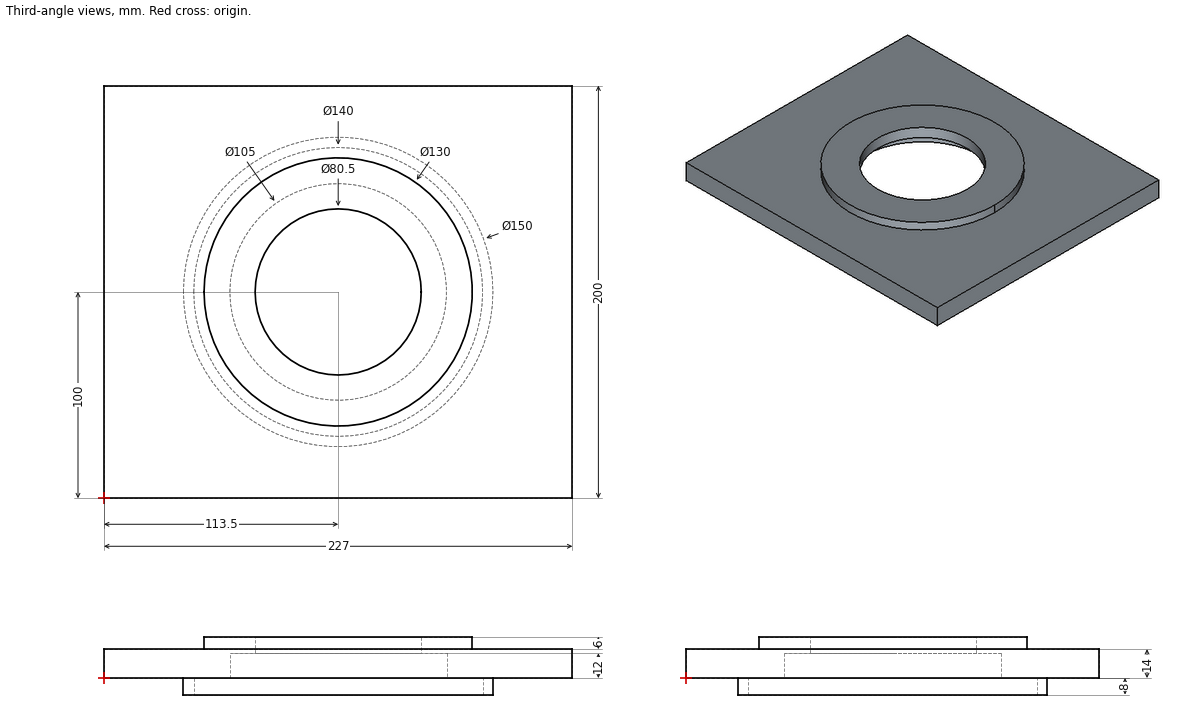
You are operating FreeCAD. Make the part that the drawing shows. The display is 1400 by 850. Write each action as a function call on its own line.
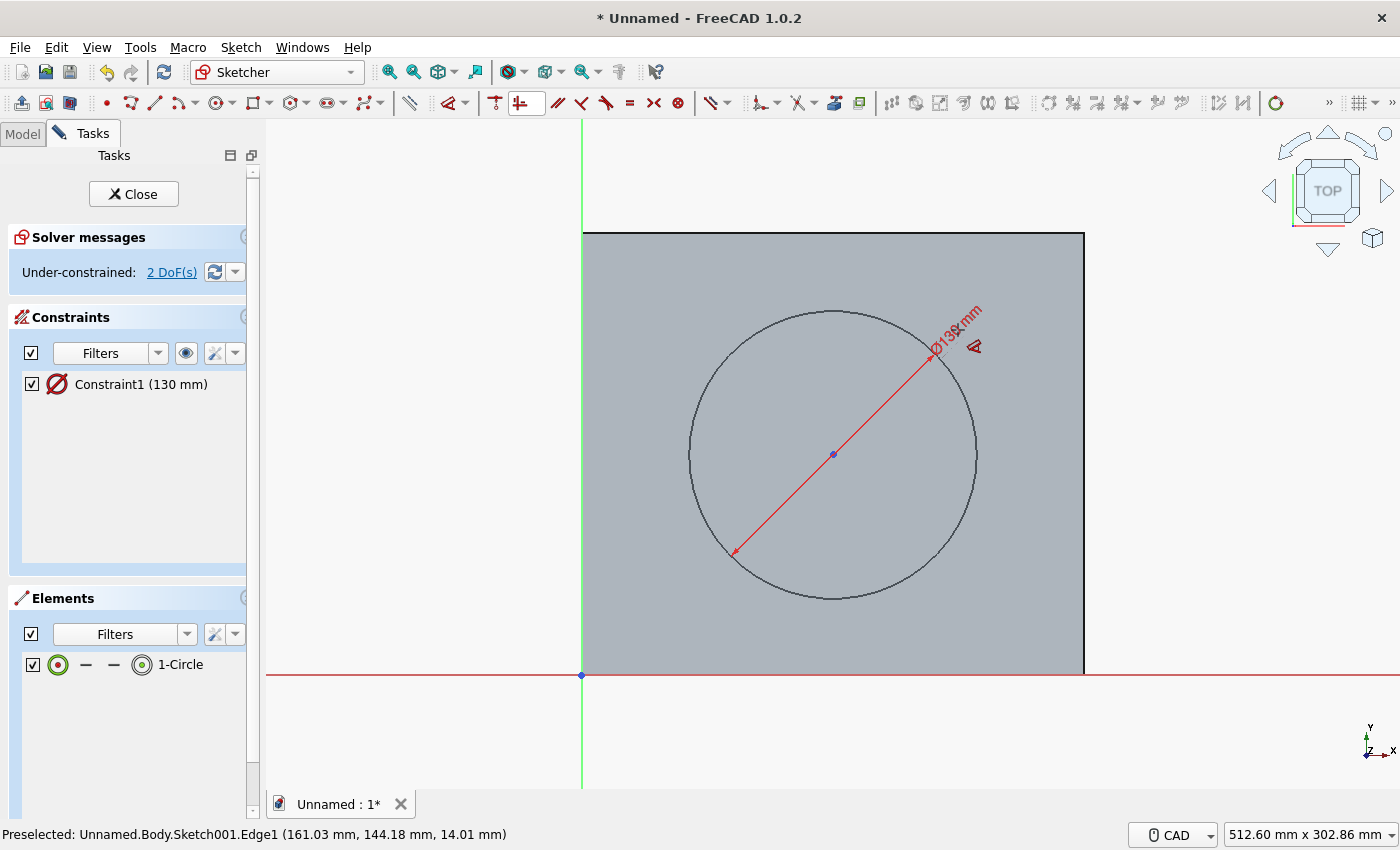
click(833, 455)
click(548, 565)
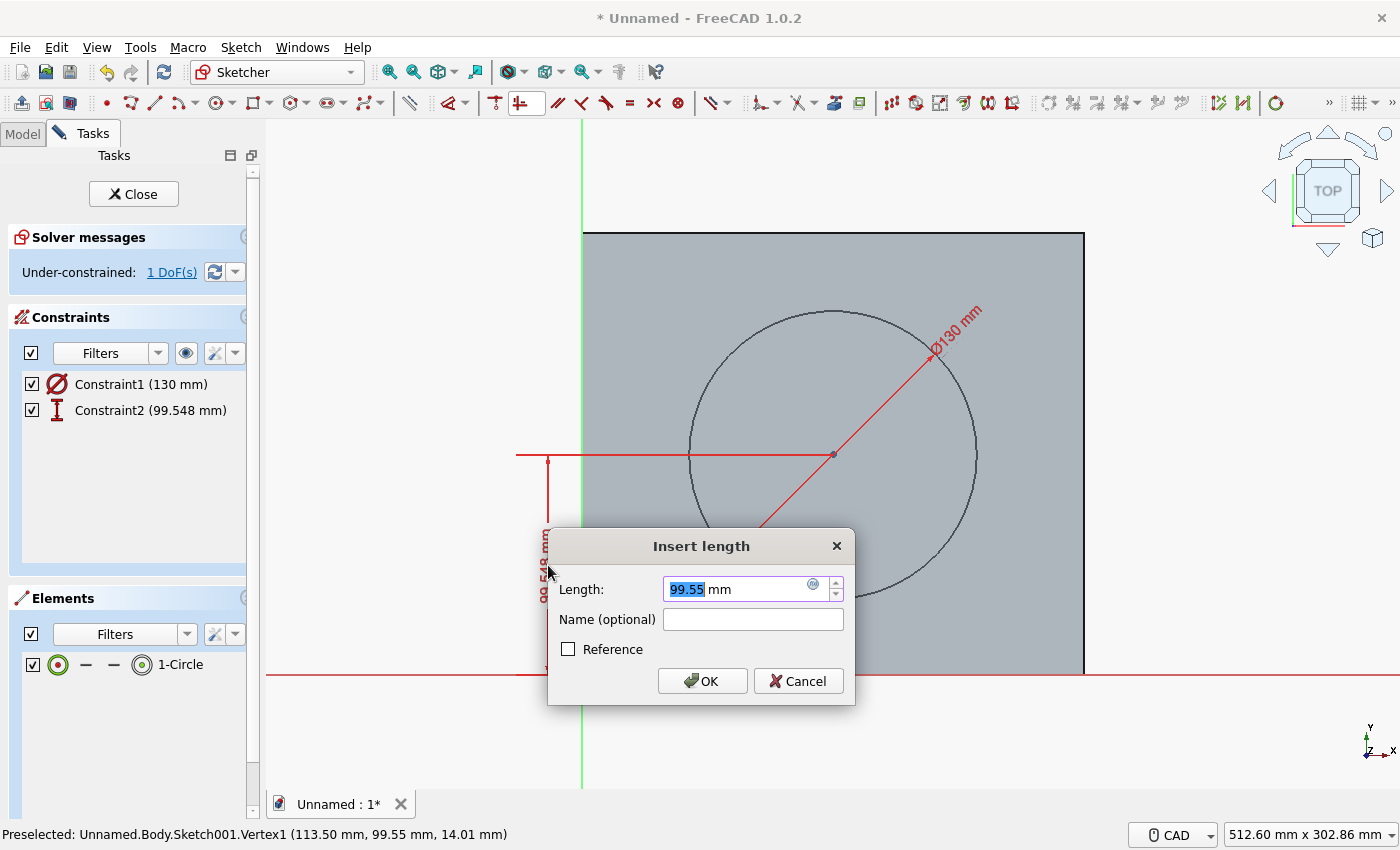
text(100)
key(Return)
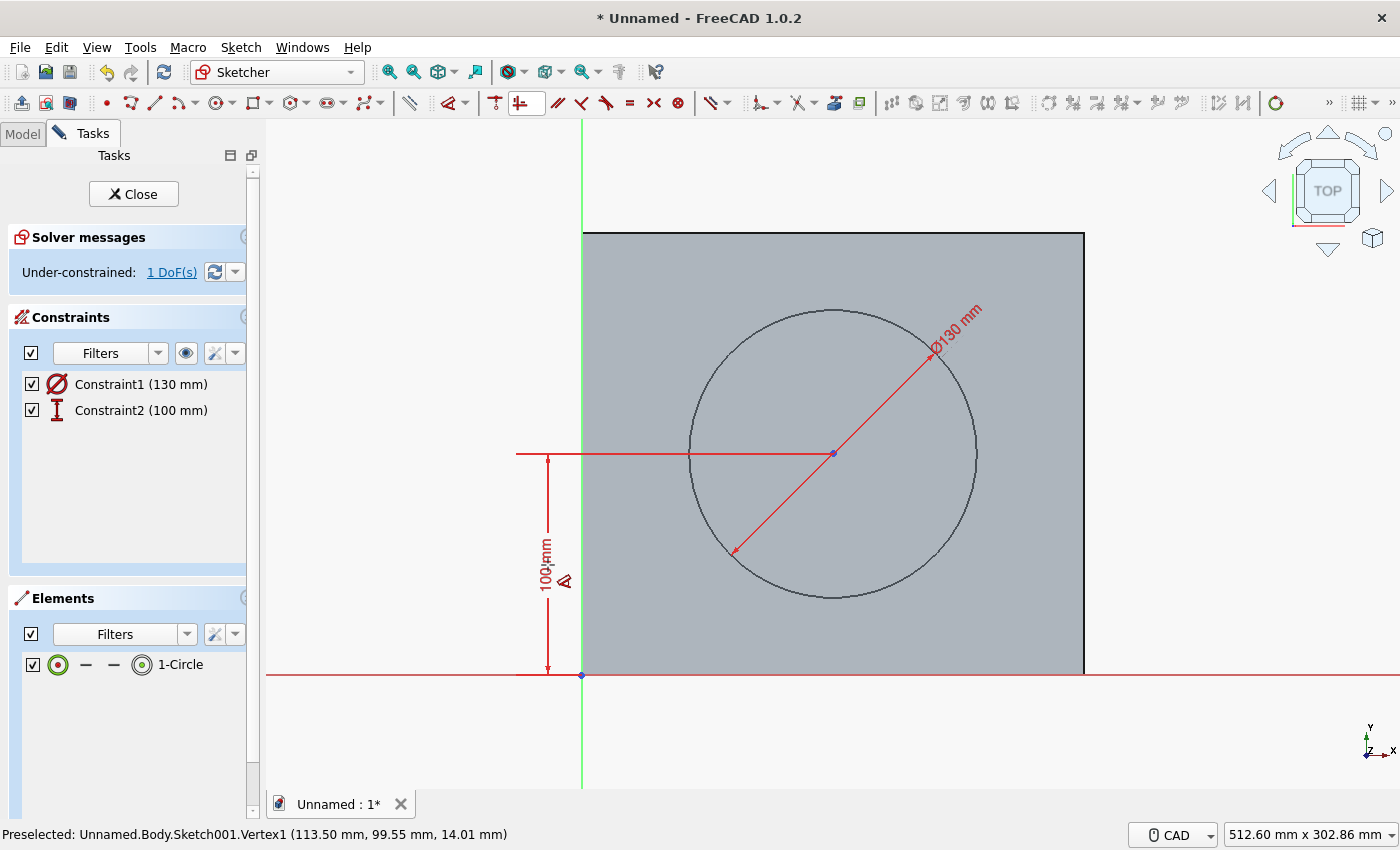
click(833, 454)
click(707, 709)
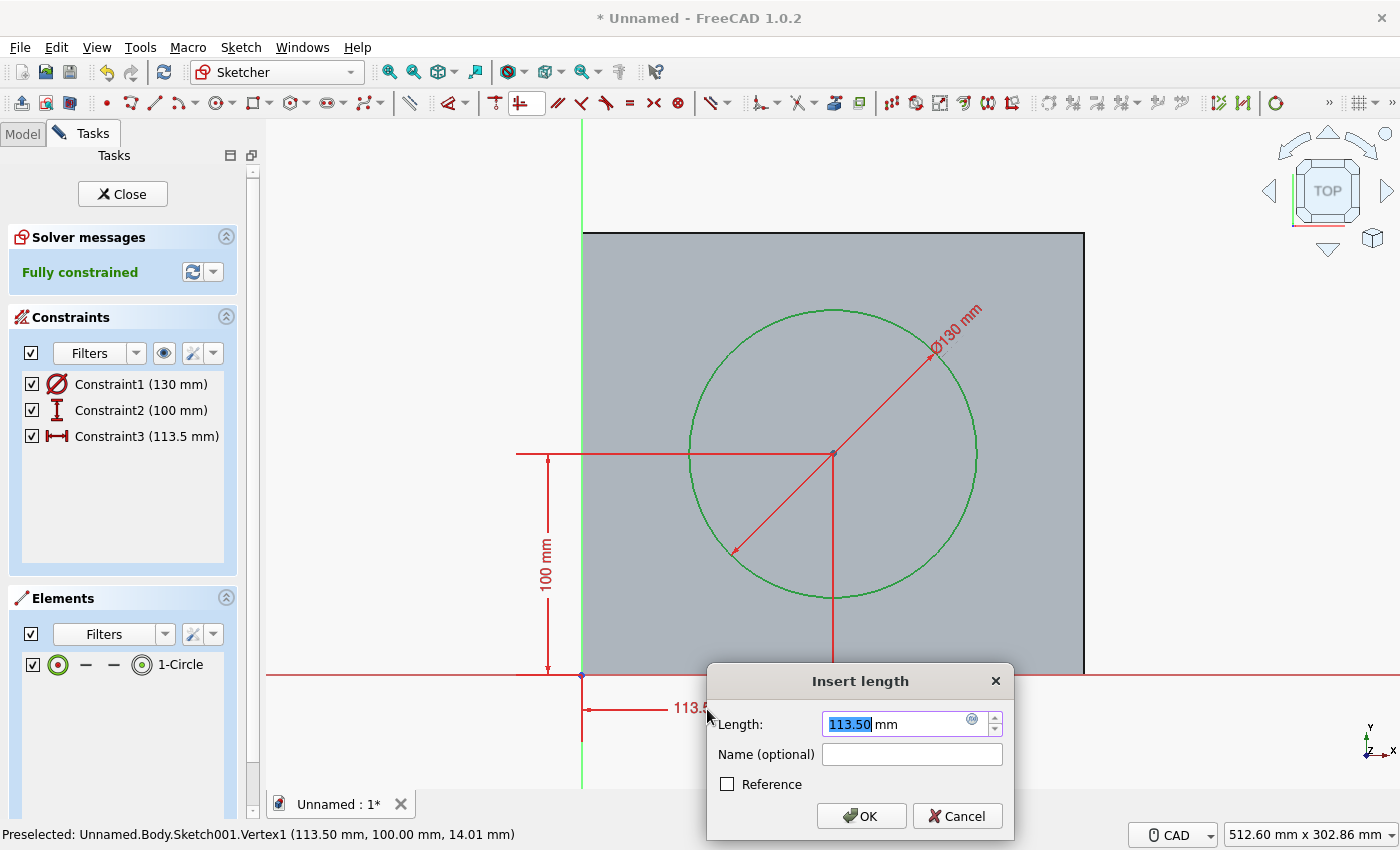
text(113.5)
key(Return)
key(Escape)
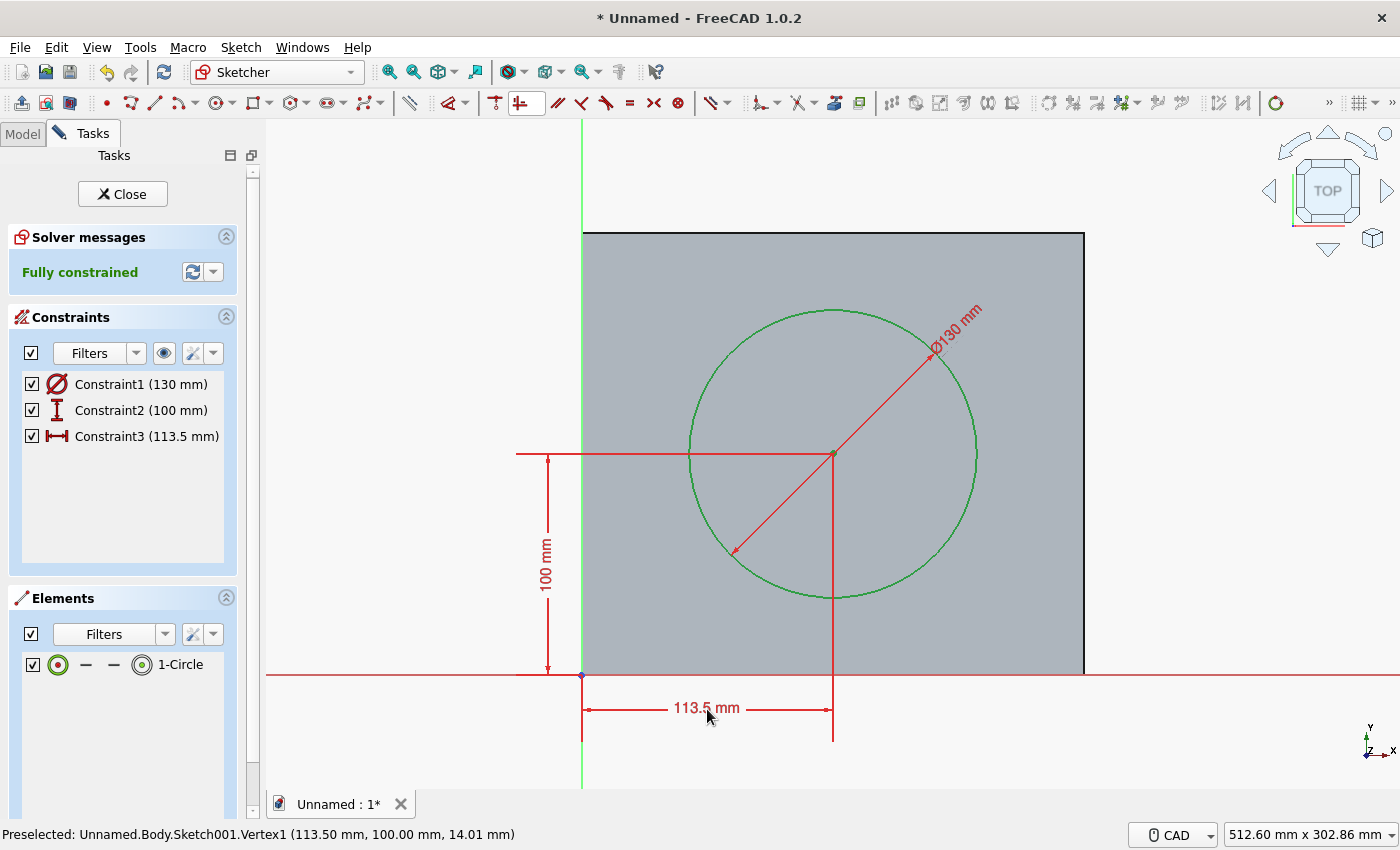
click(123, 194)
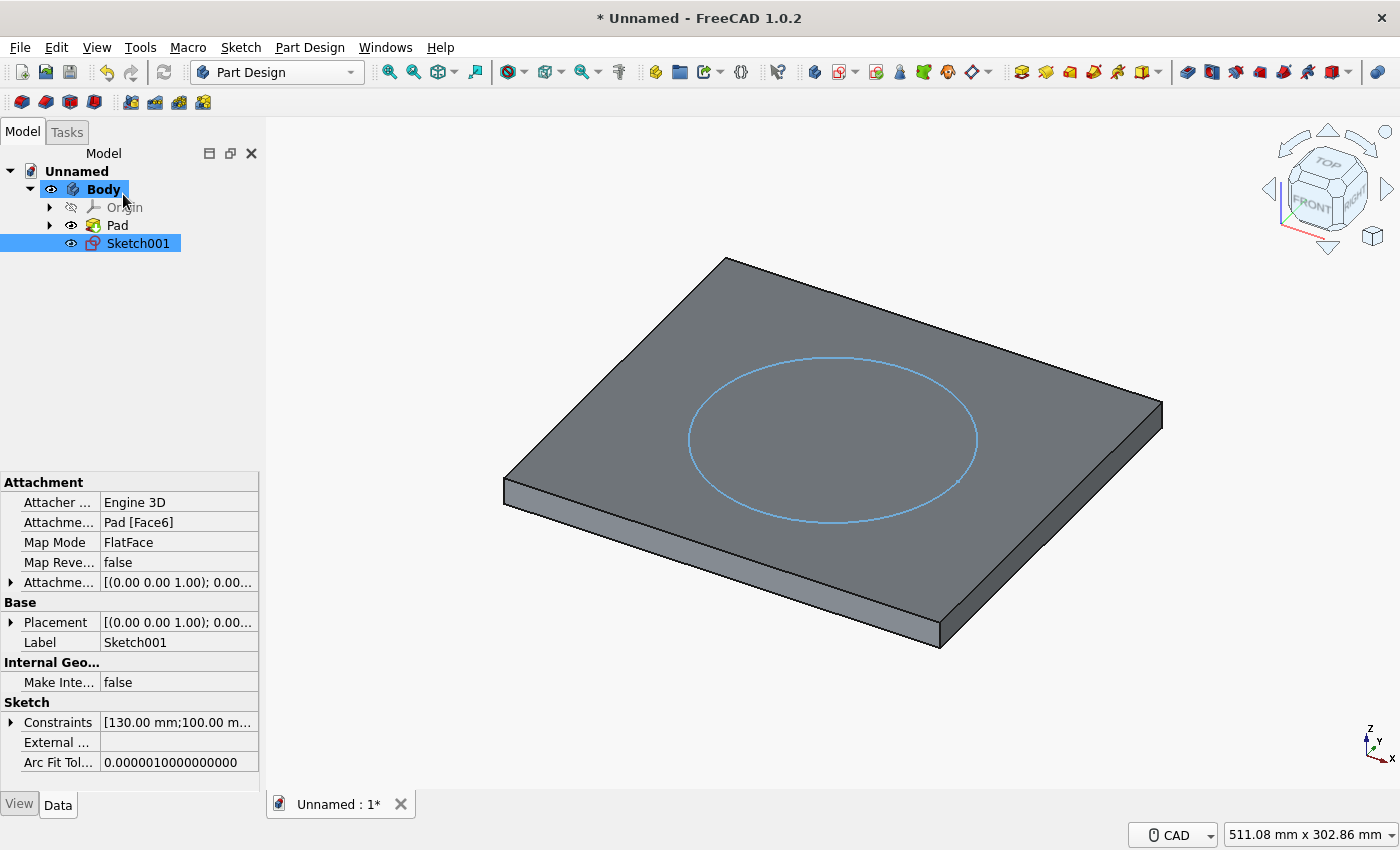
click(1022, 72)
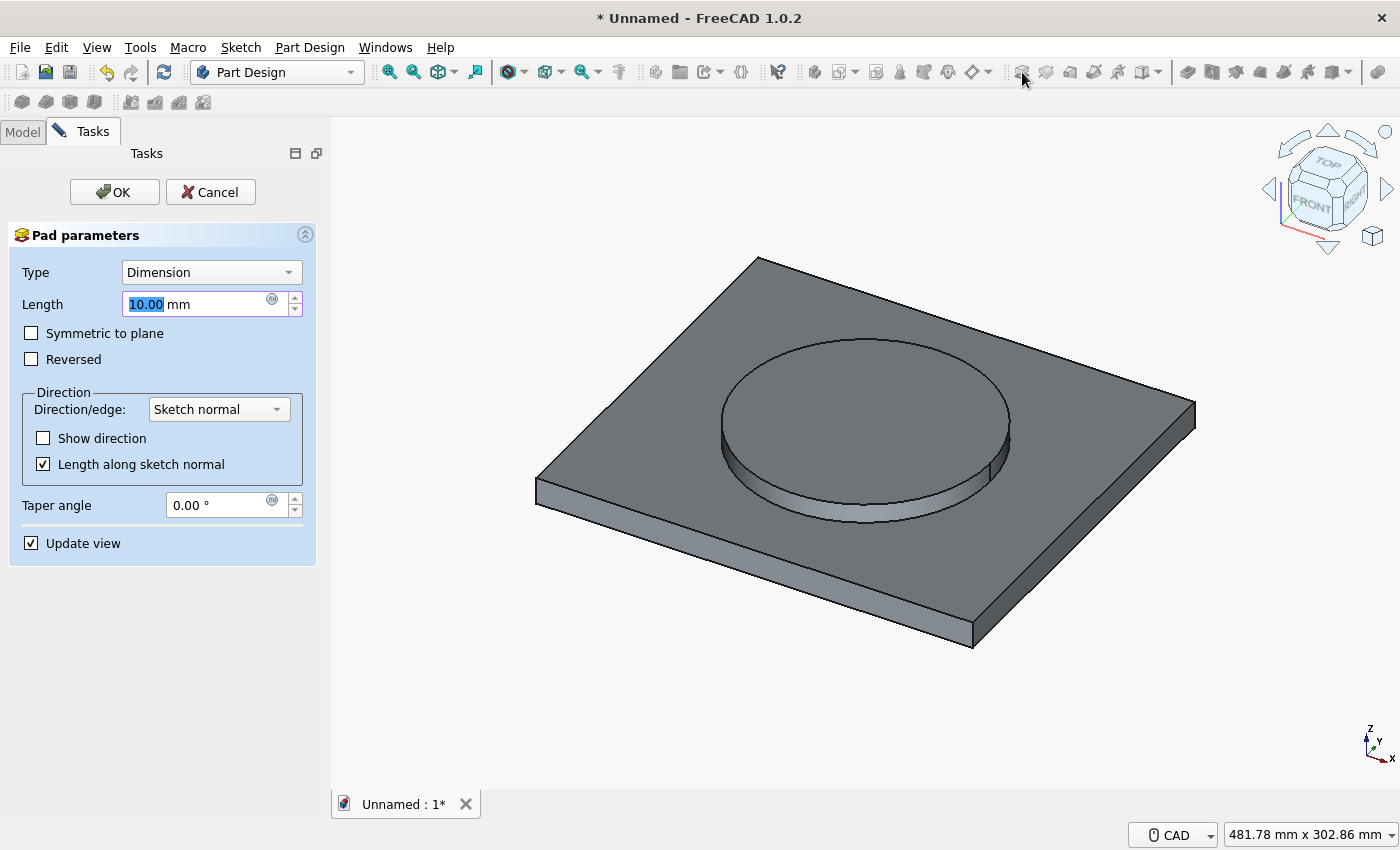
text(6)
key(Tab)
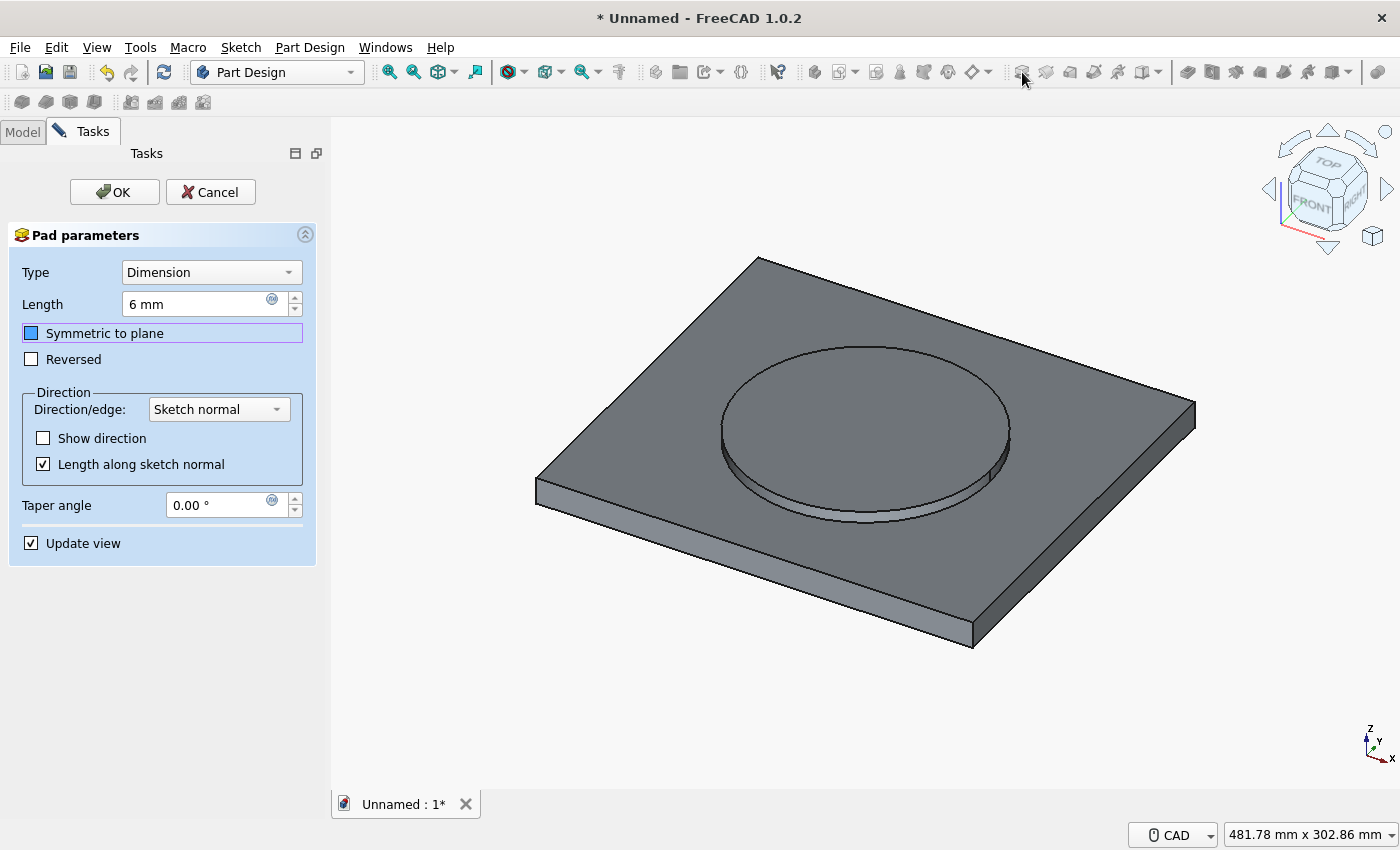
click(115, 192)